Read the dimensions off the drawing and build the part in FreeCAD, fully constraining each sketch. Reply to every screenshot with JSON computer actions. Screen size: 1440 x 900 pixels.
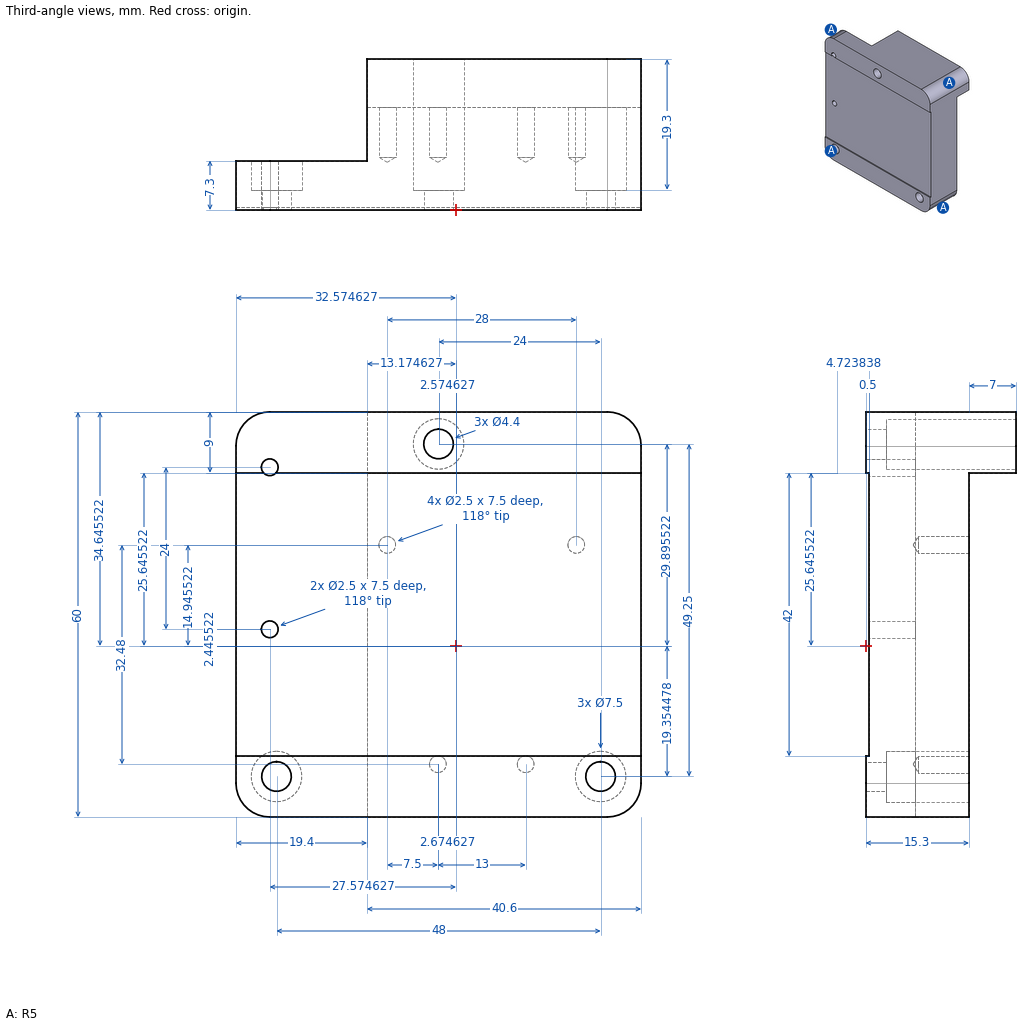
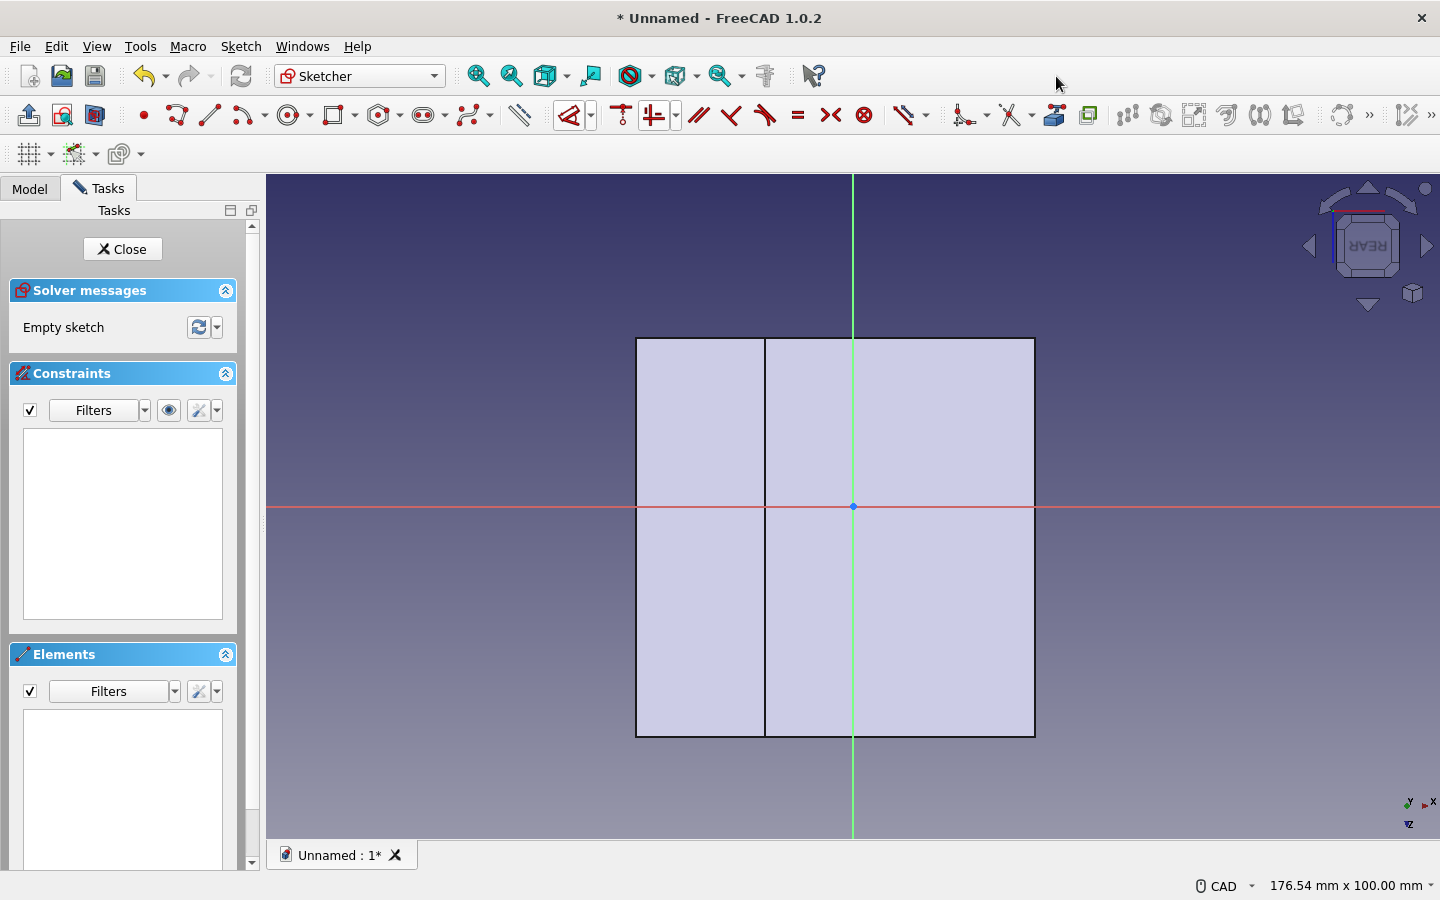
{"action": "scroll", "coordinate": [1041, 762], "scroll_direction": "up", "scroll_amount": 3}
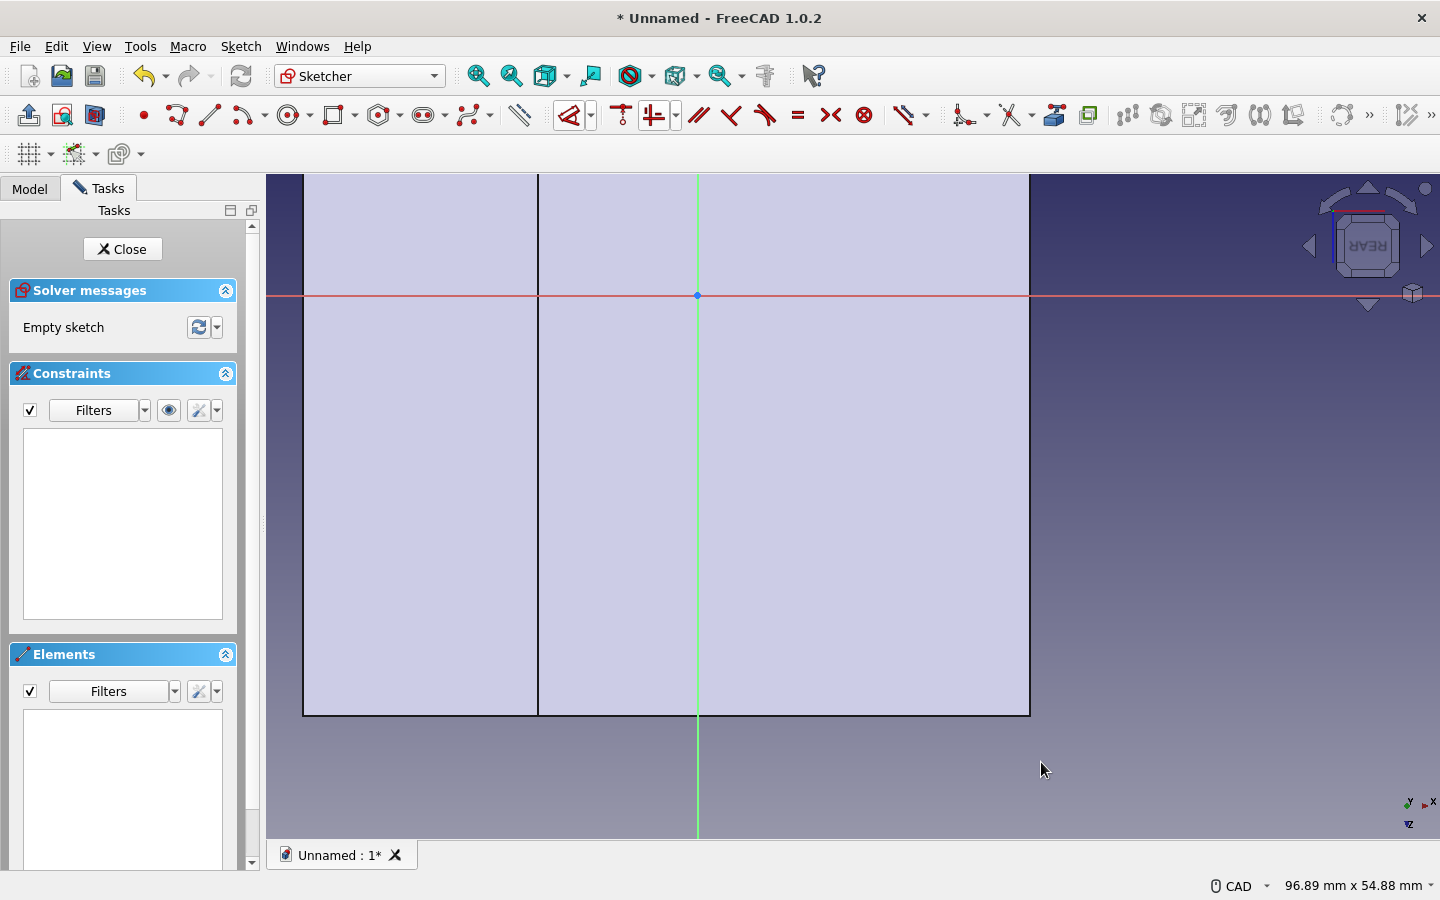
{"action": "key", "text": "g r"}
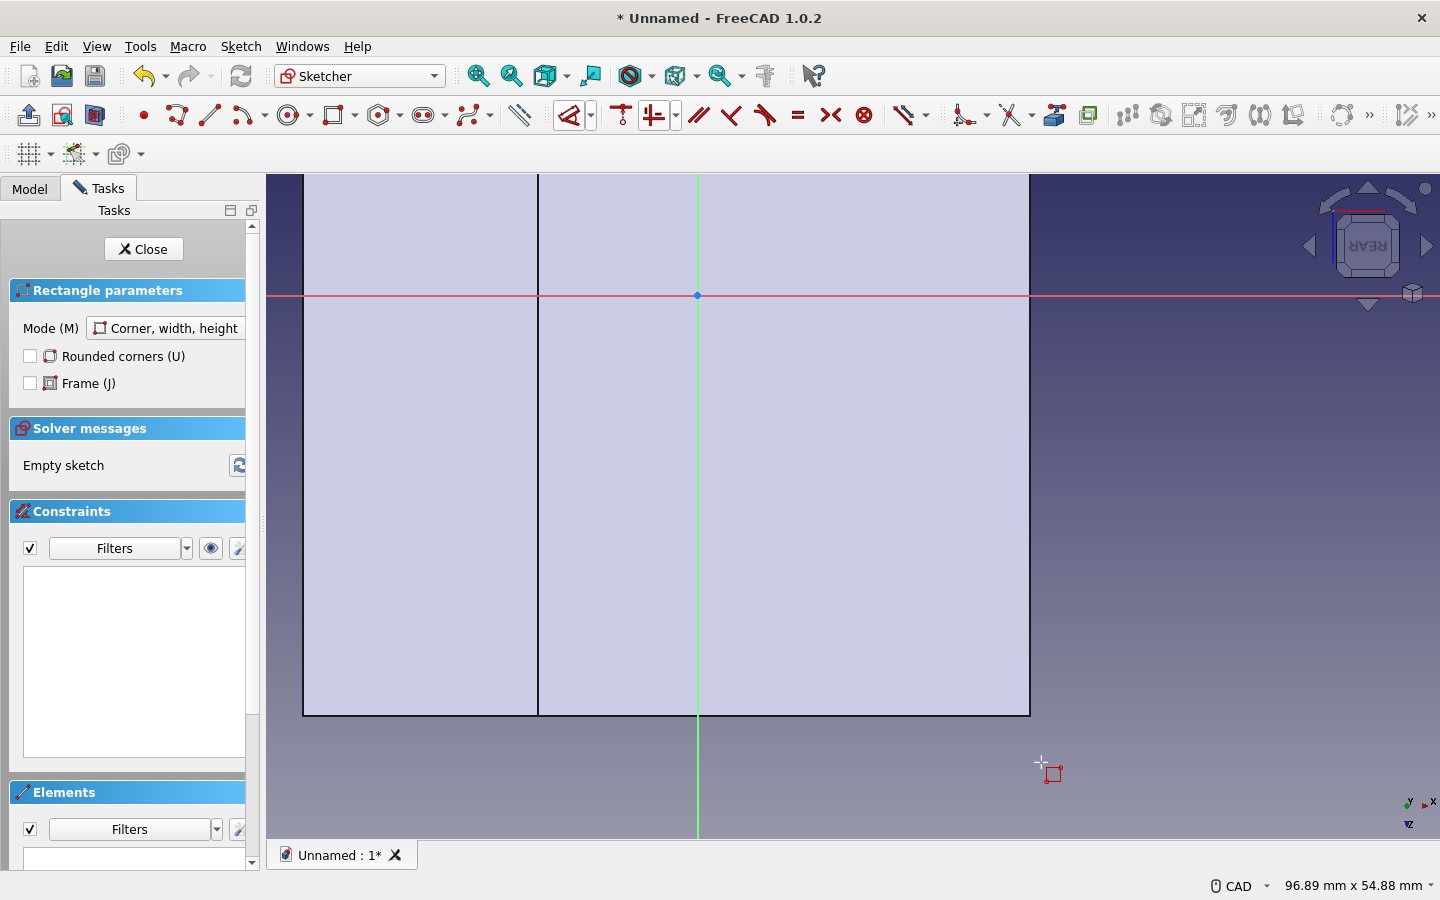
{"action": "left_click", "coordinate": [538, 606]}
{"action": "left_click", "coordinate": [1030, 716]}
{"action": "key", "text": "Escape"}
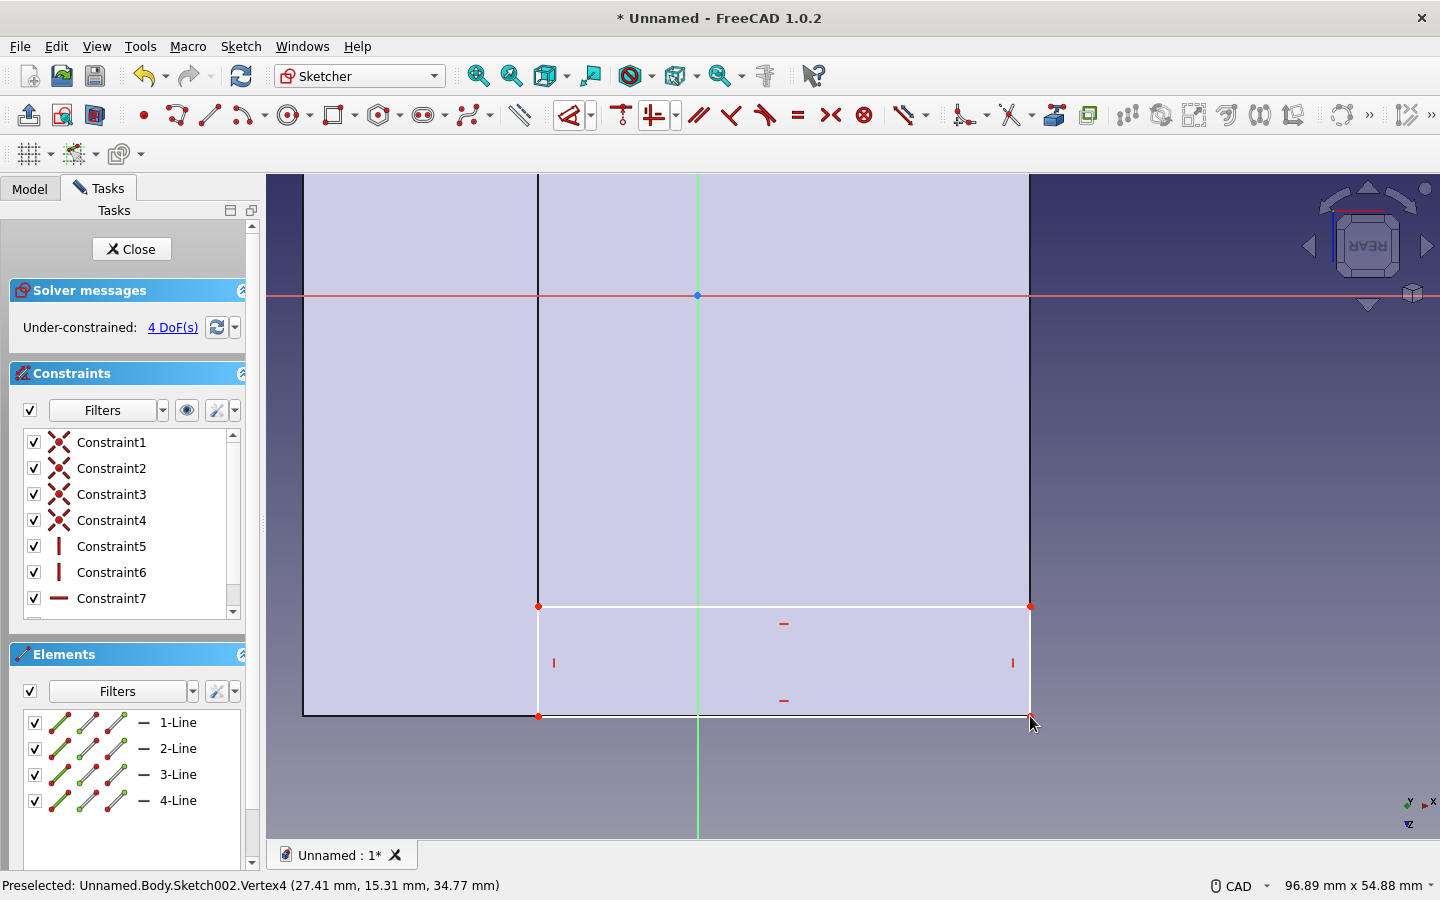
{"action": "left_click", "coordinate": [568, 116]}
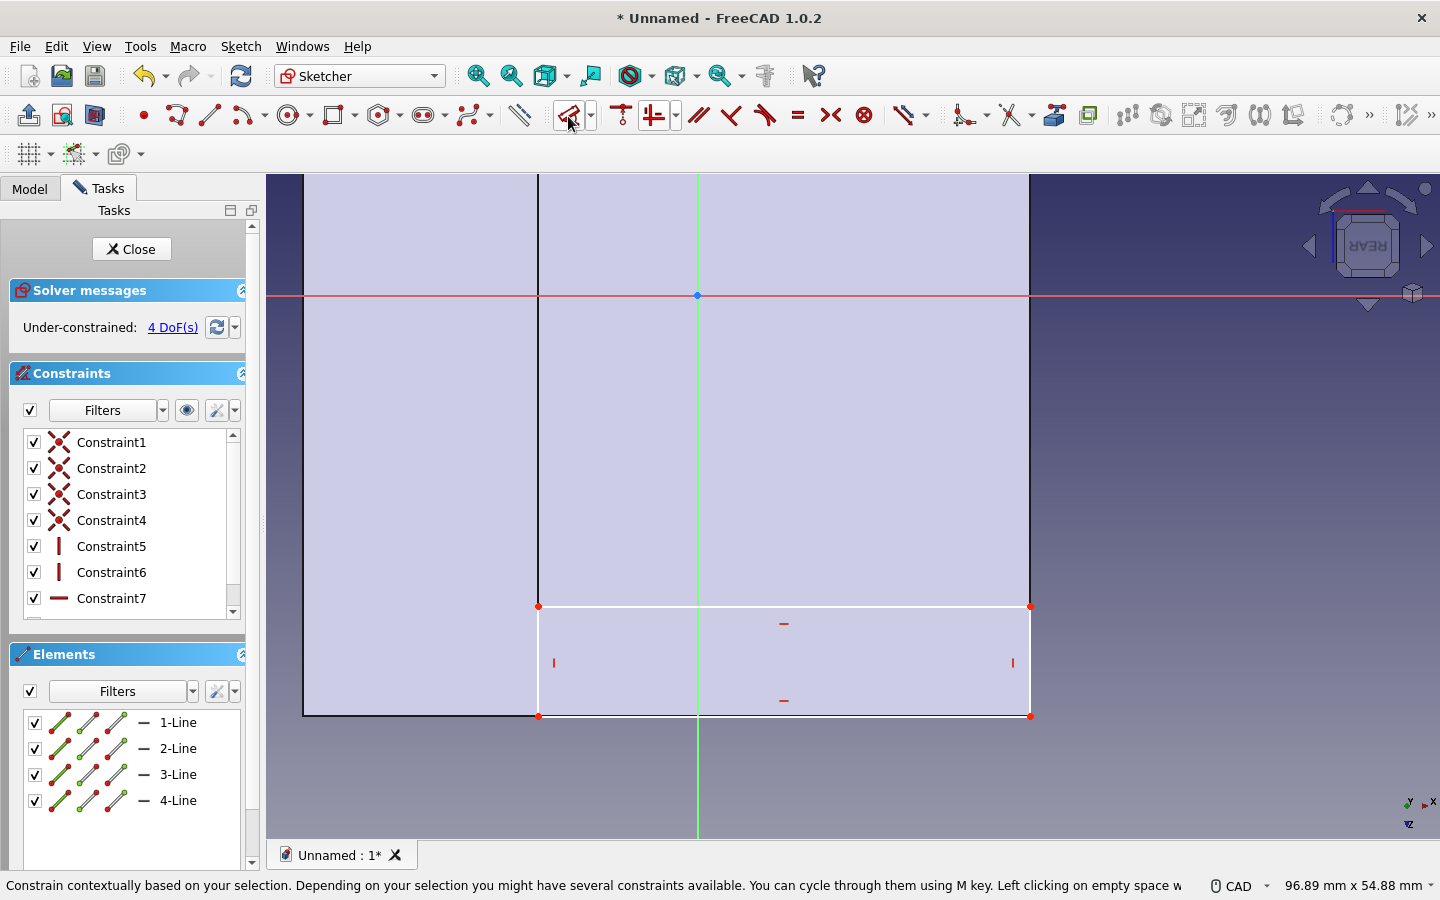
{"action": "left_click", "coordinate": [538, 640]}
{"action": "left_click", "coordinate": [504, 662]}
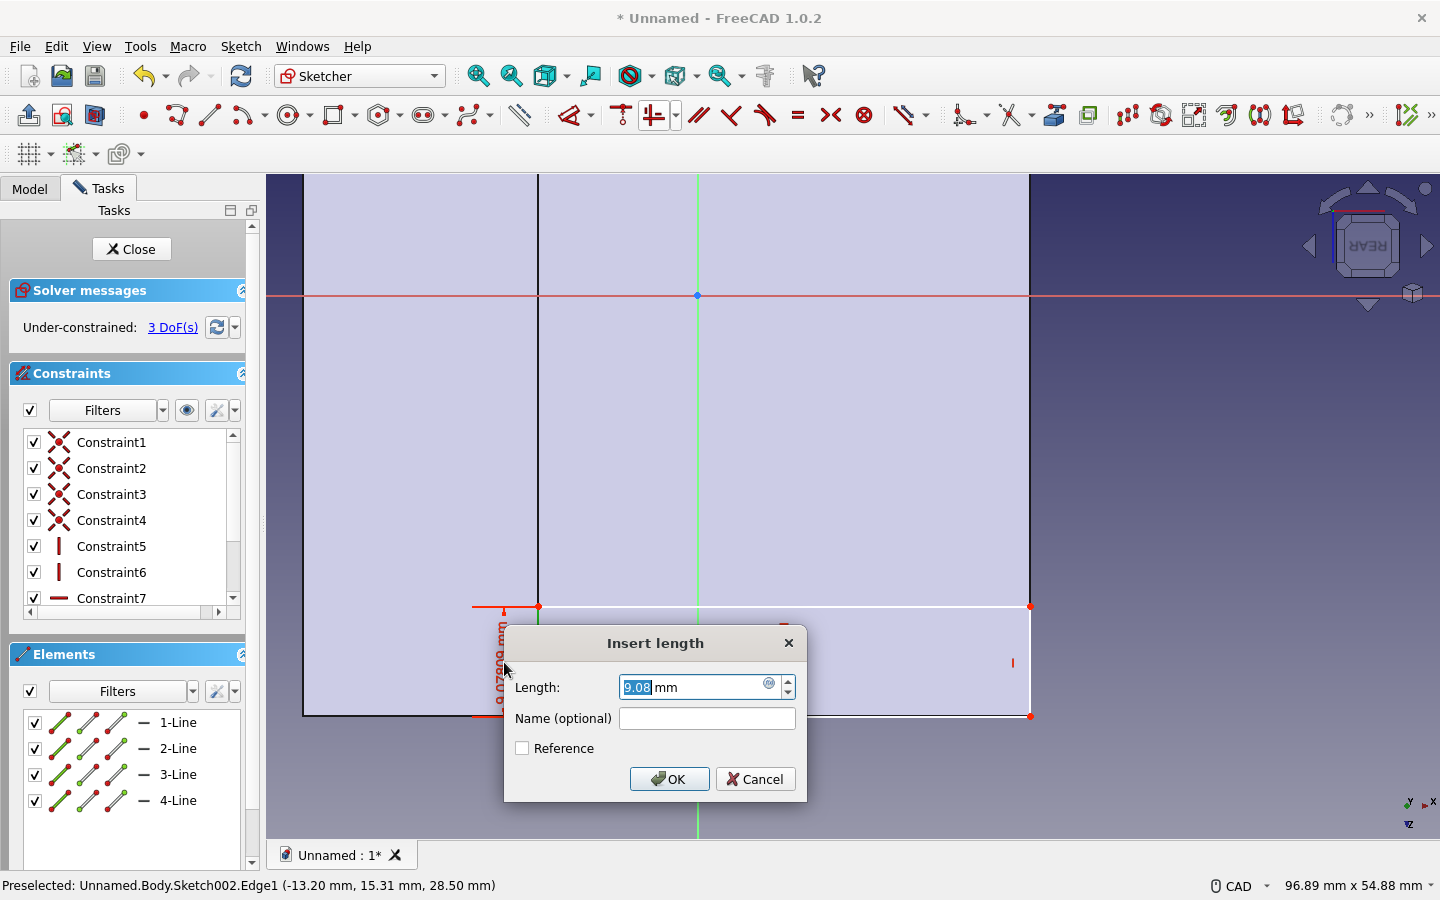
{"action": "type", "text": "9"}
{"action": "key", "text": "Return"}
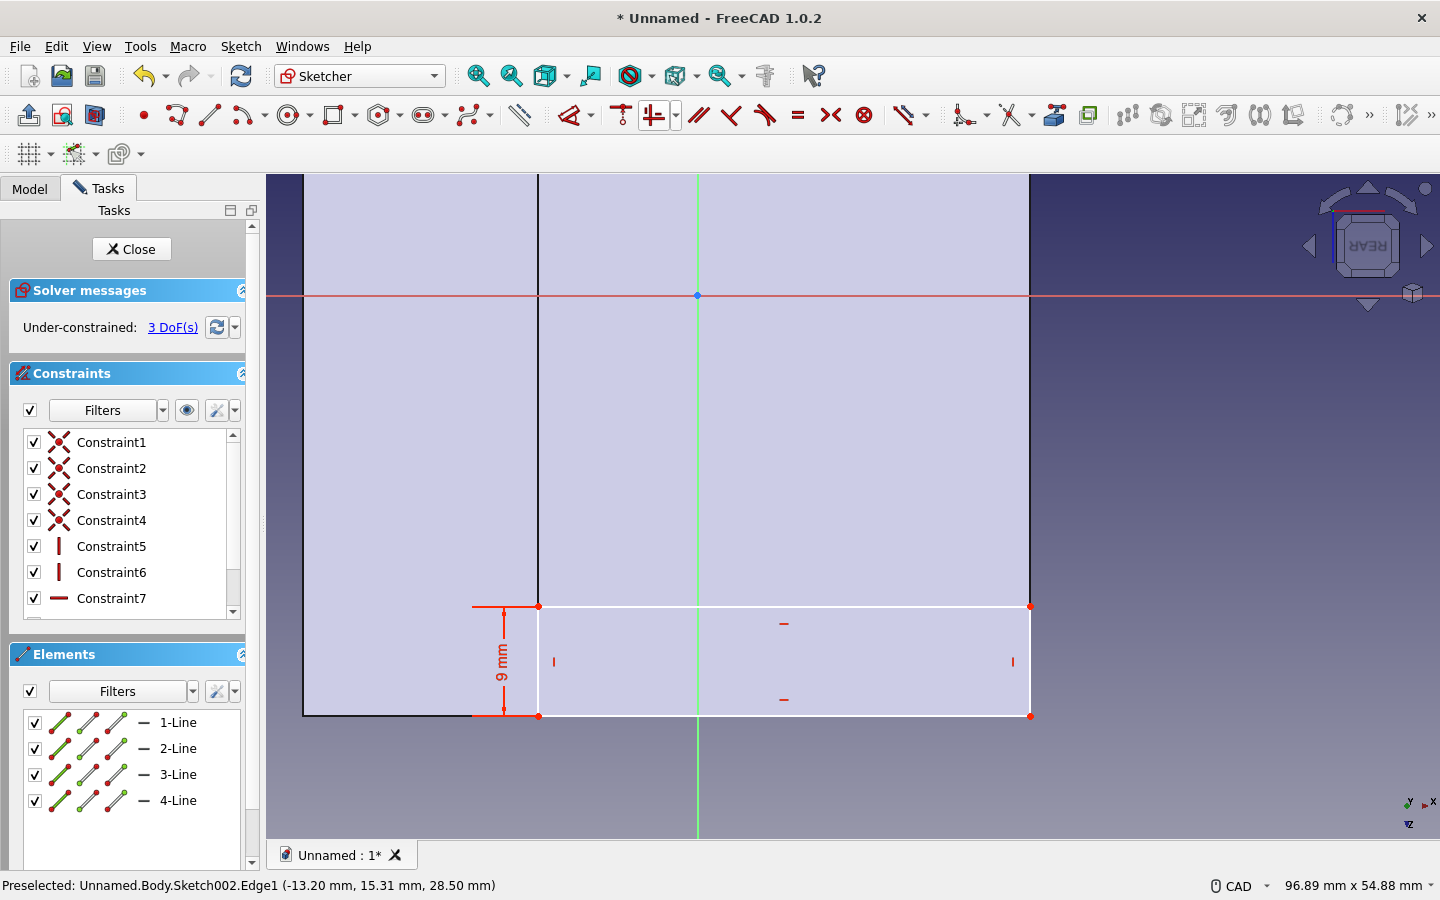
{"action": "left_click", "coordinate": [686, 716]}
{"action": "left_click", "coordinate": [784, 750]}